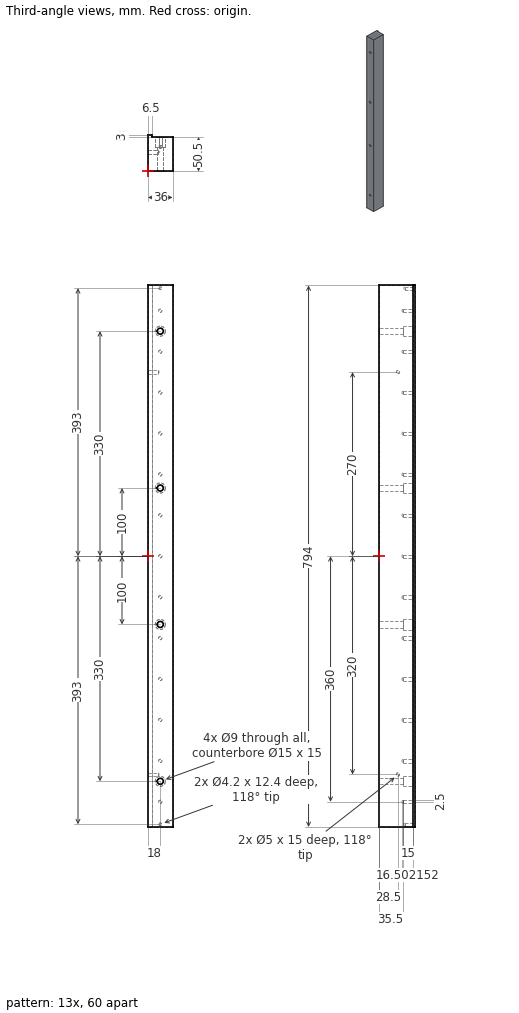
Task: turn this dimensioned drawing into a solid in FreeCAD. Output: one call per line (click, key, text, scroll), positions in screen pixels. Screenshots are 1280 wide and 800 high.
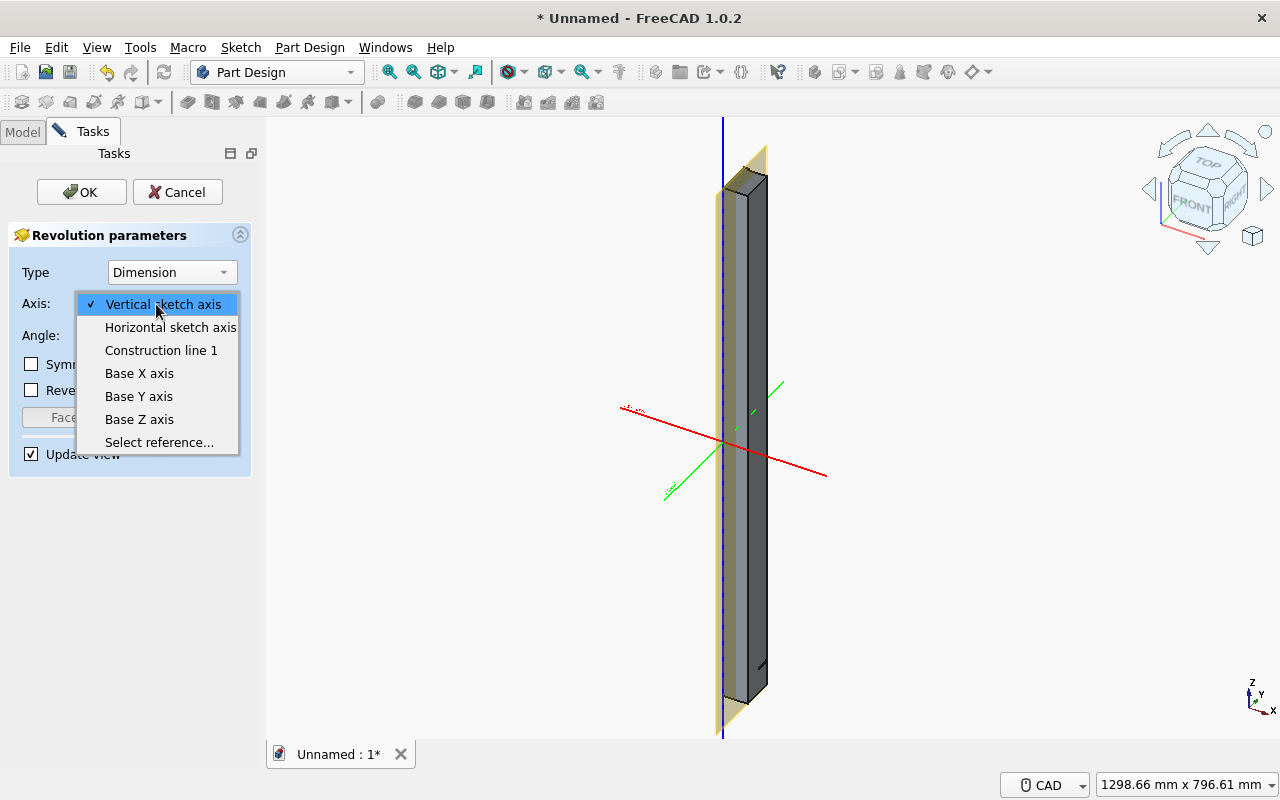
click(156, 350)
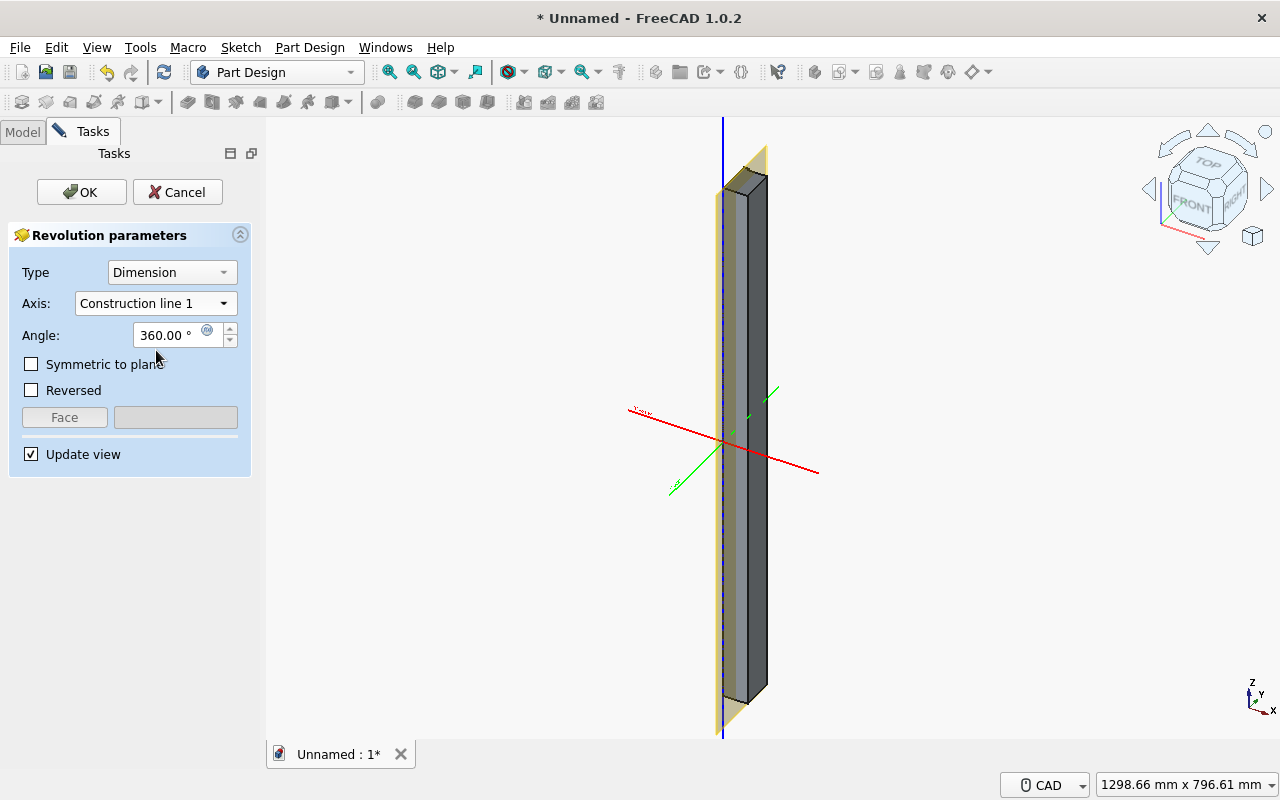
click(82, 192)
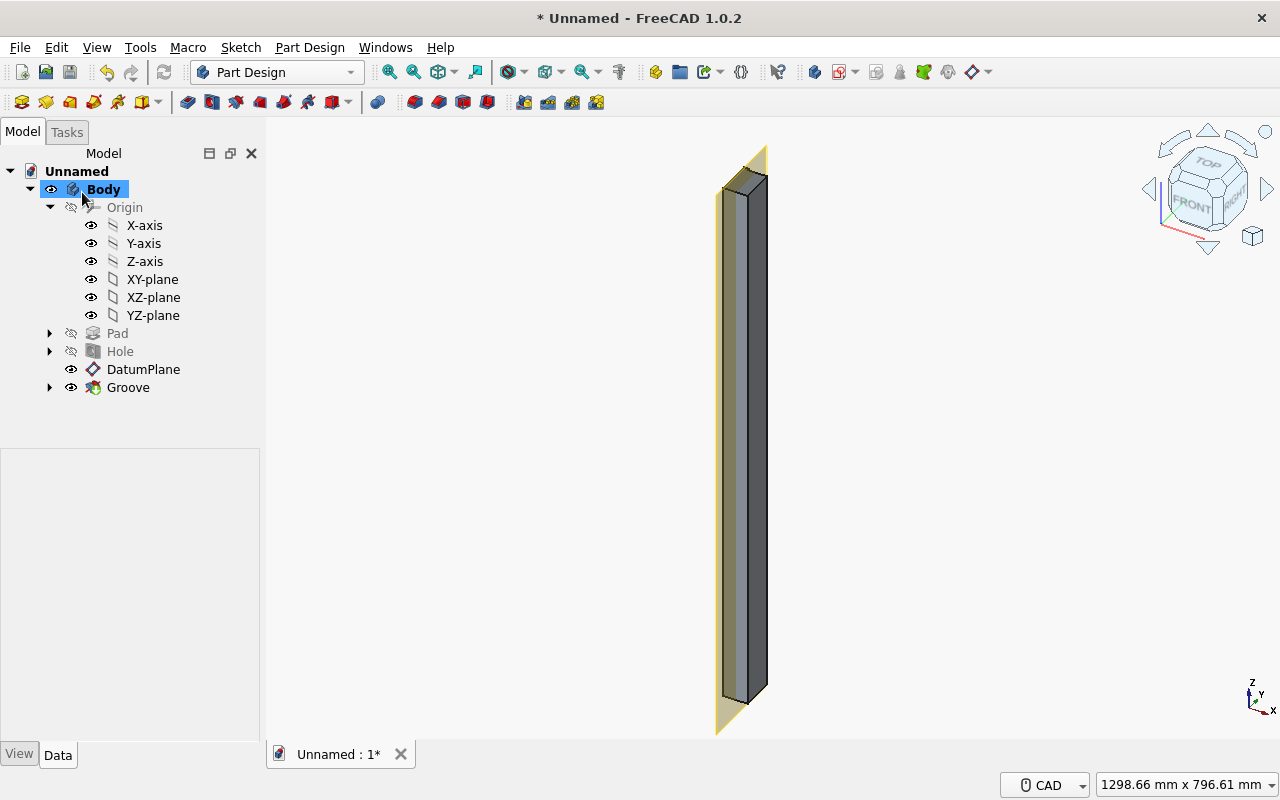
click(116, 369)
key(space)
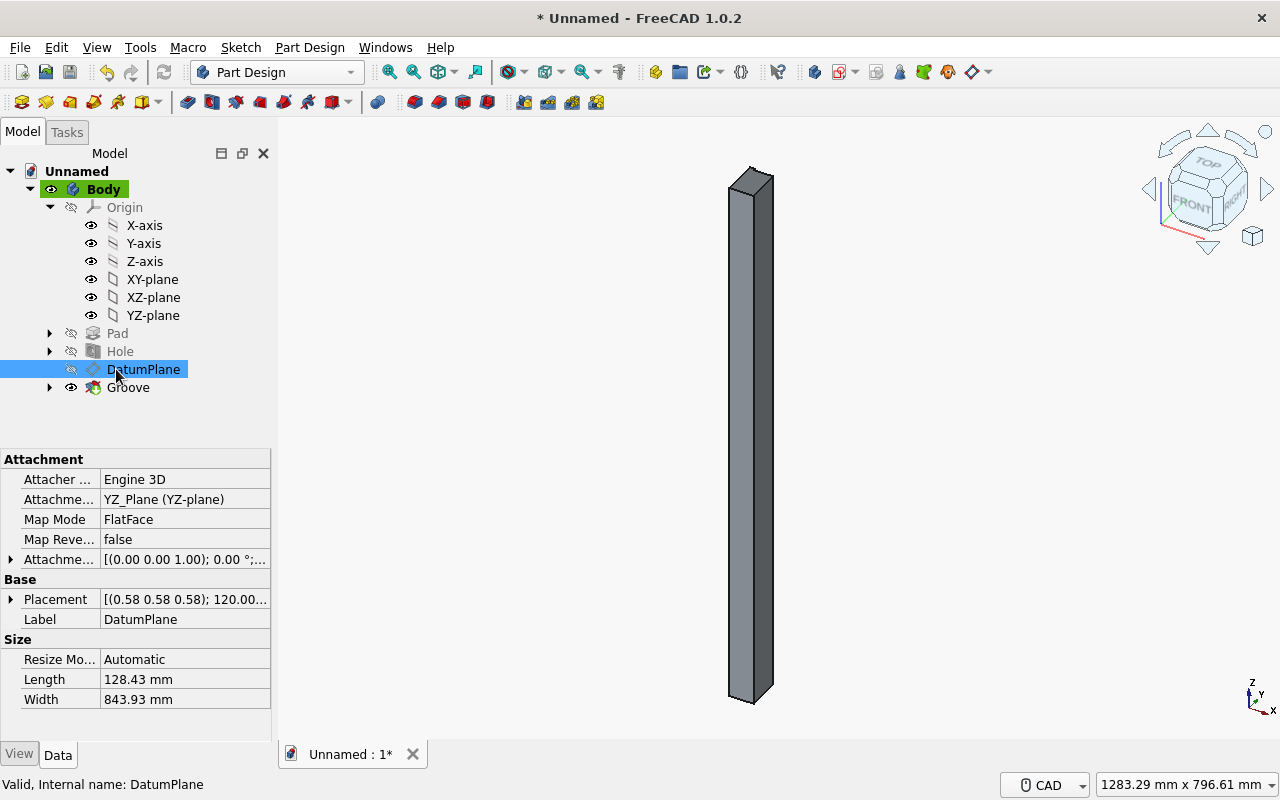
click(116, 387)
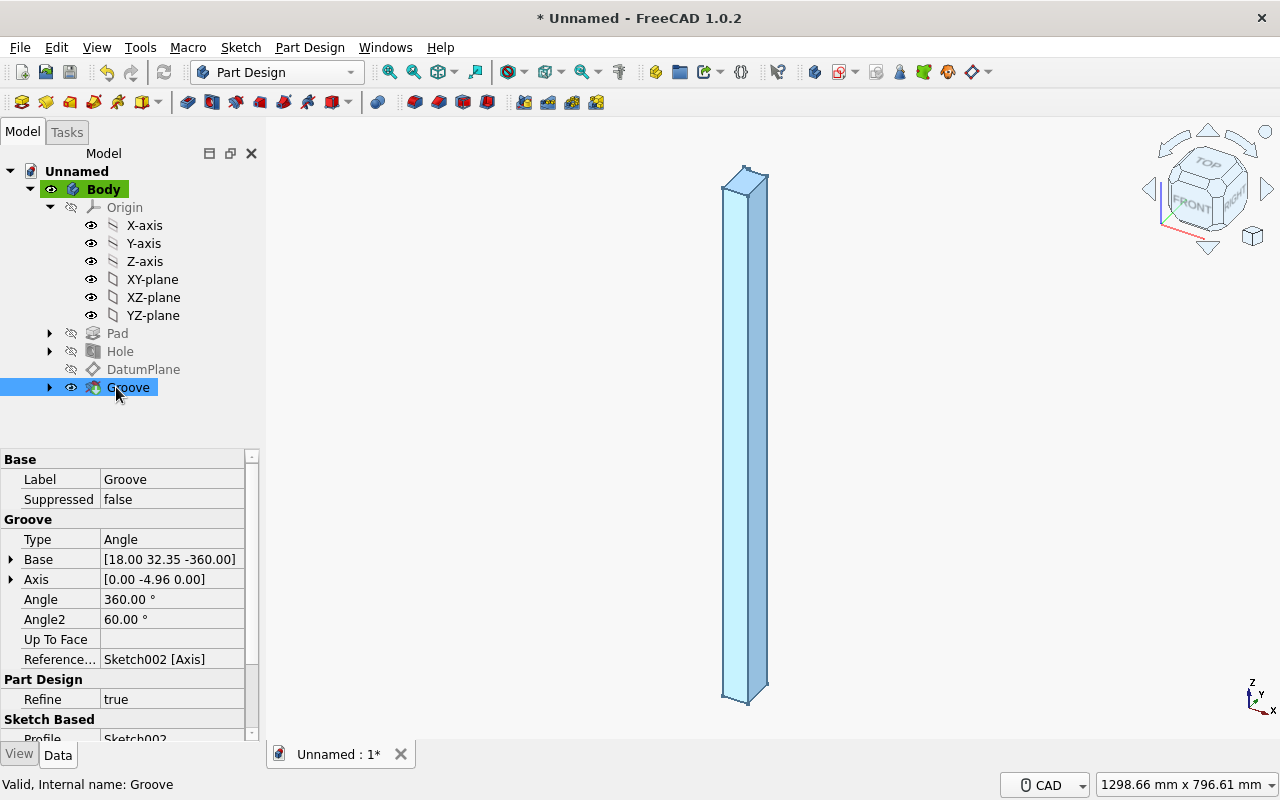
click(548, 102)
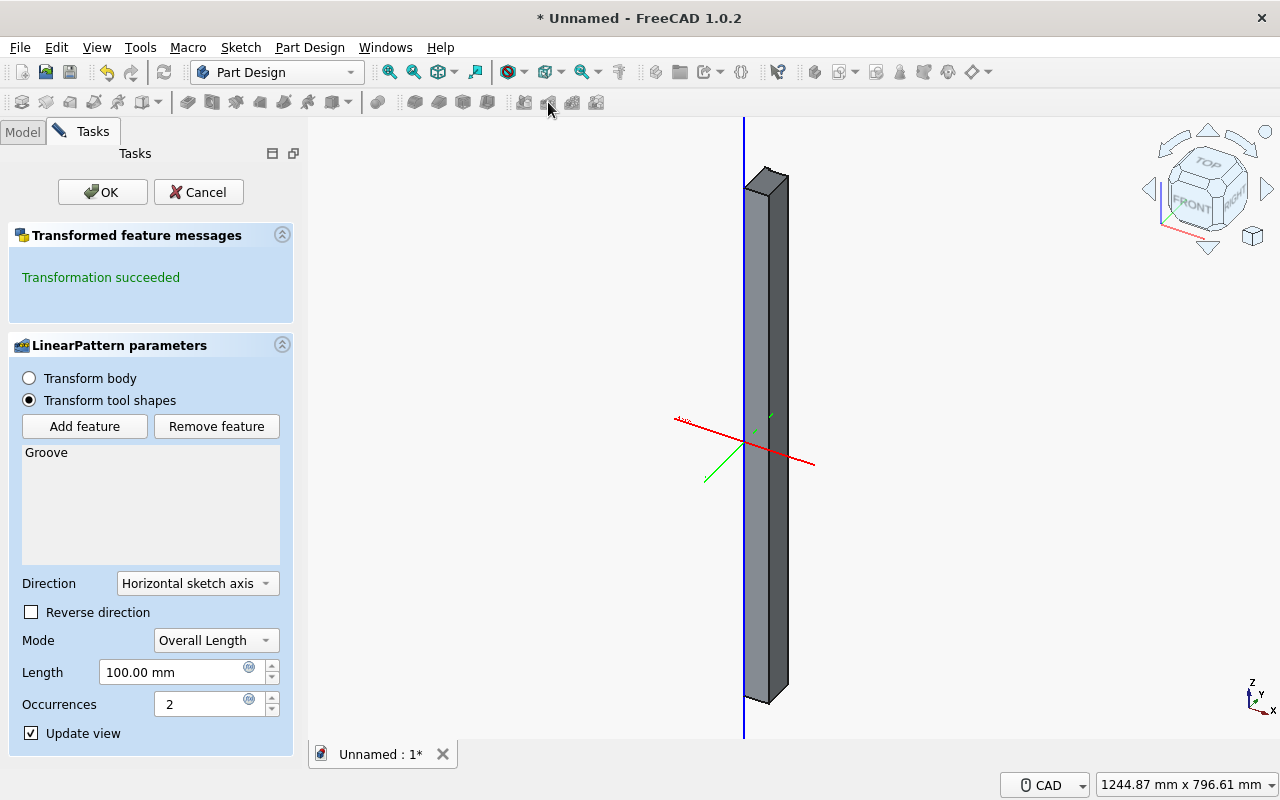
click(198, 584)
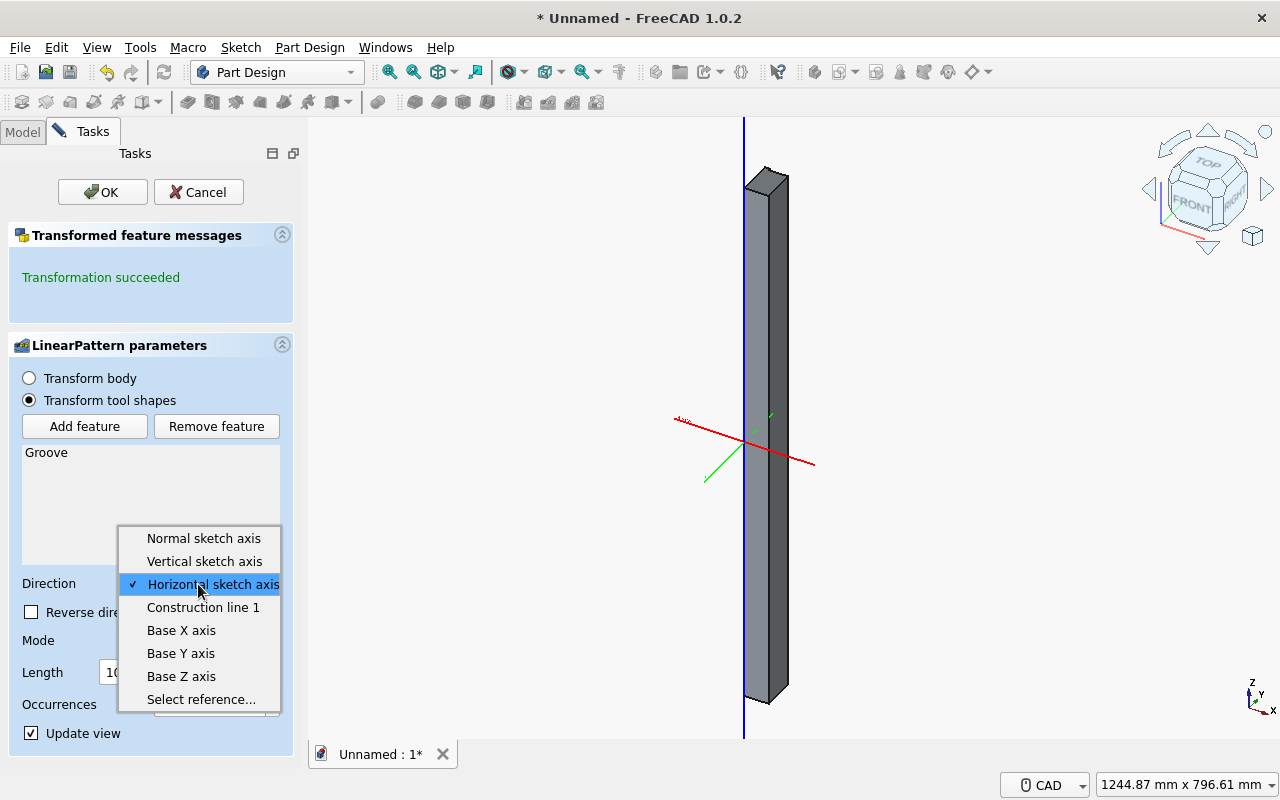
click(198, 676)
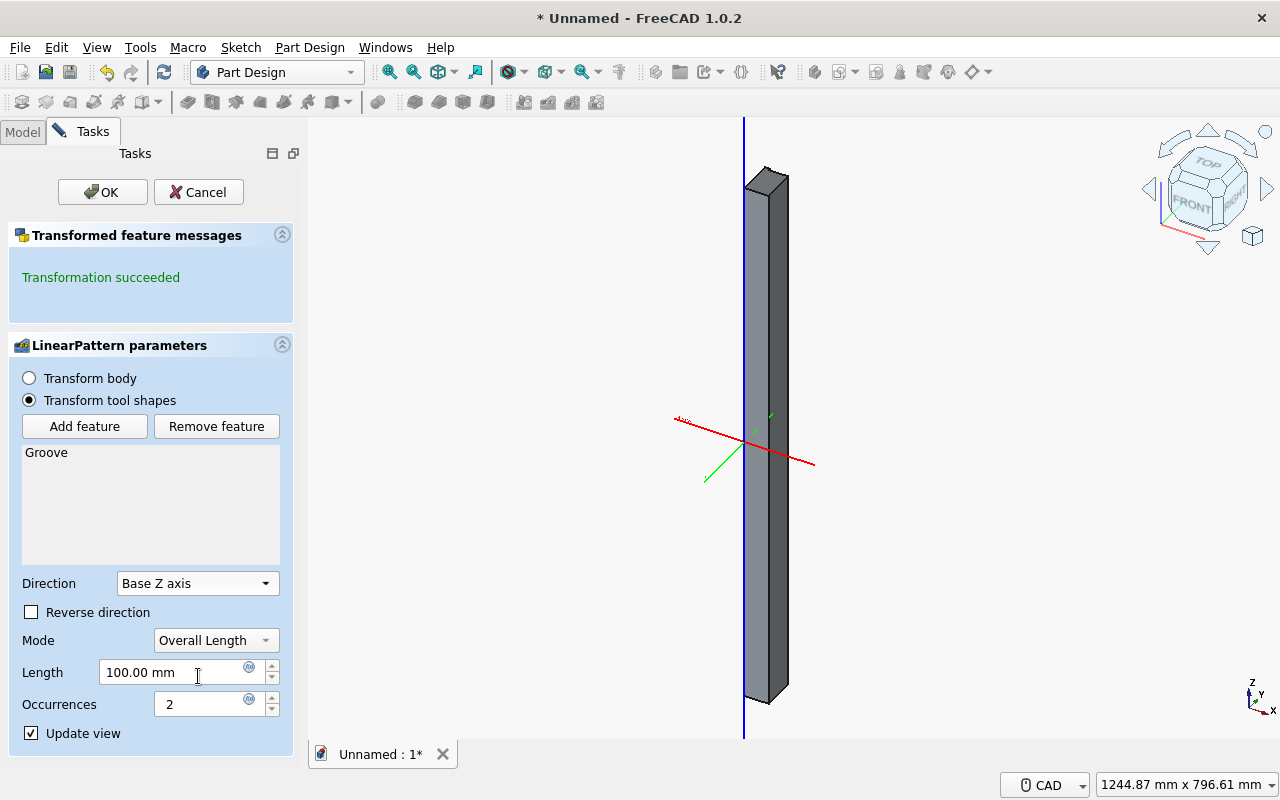
click(217, 640)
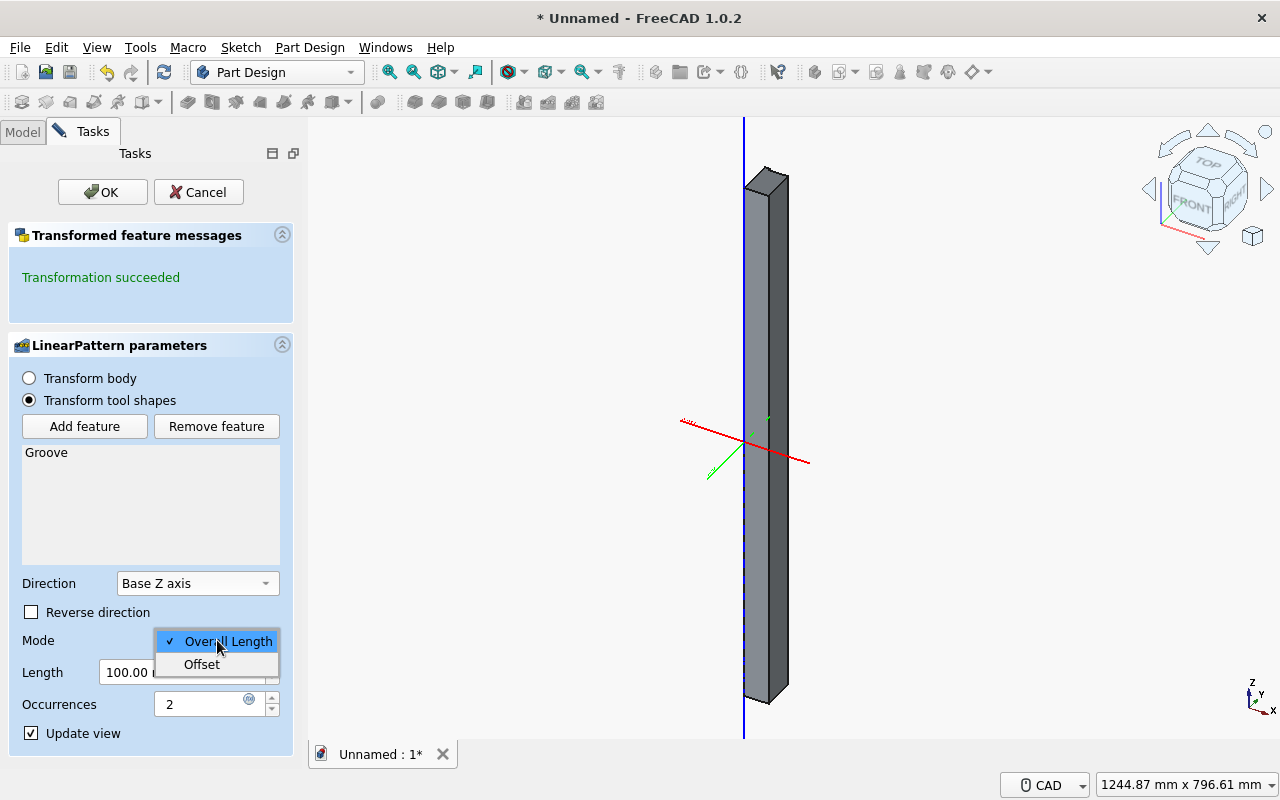
click(216, 664)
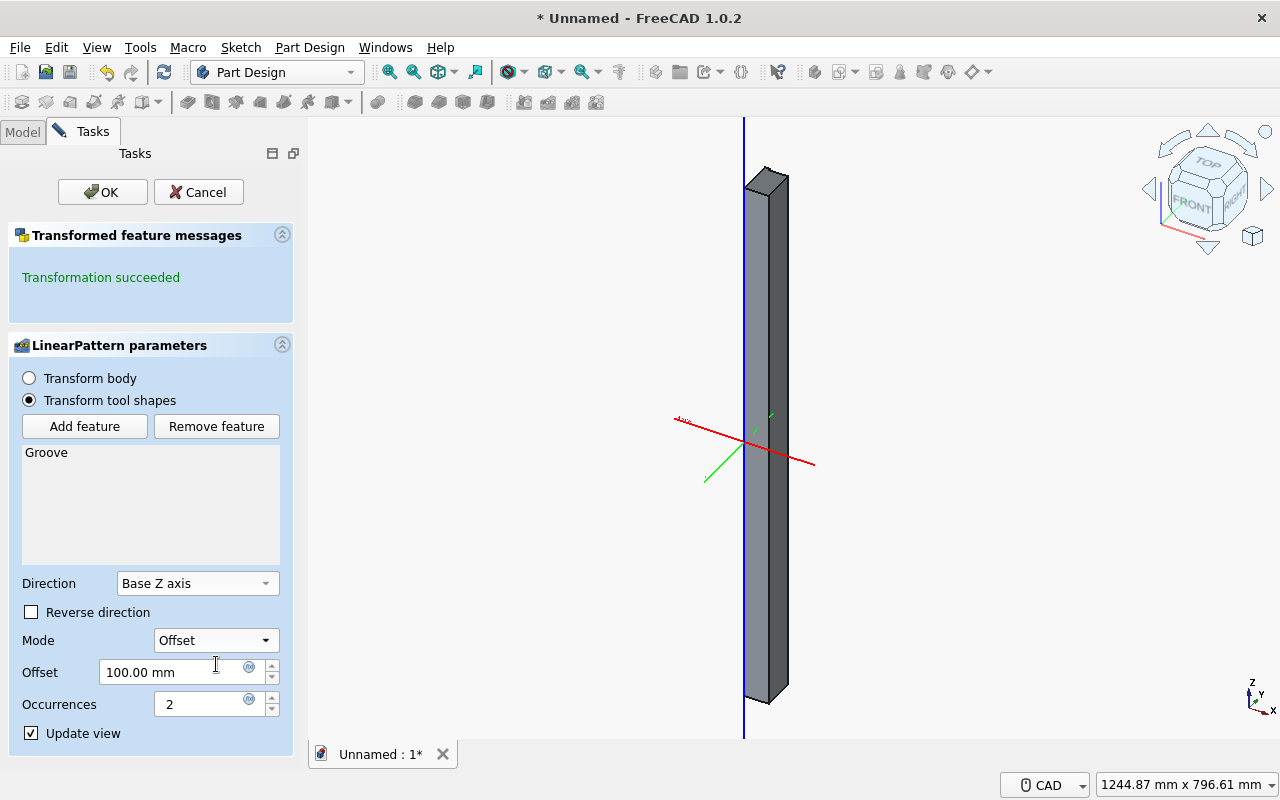
triple_click(182, 672)